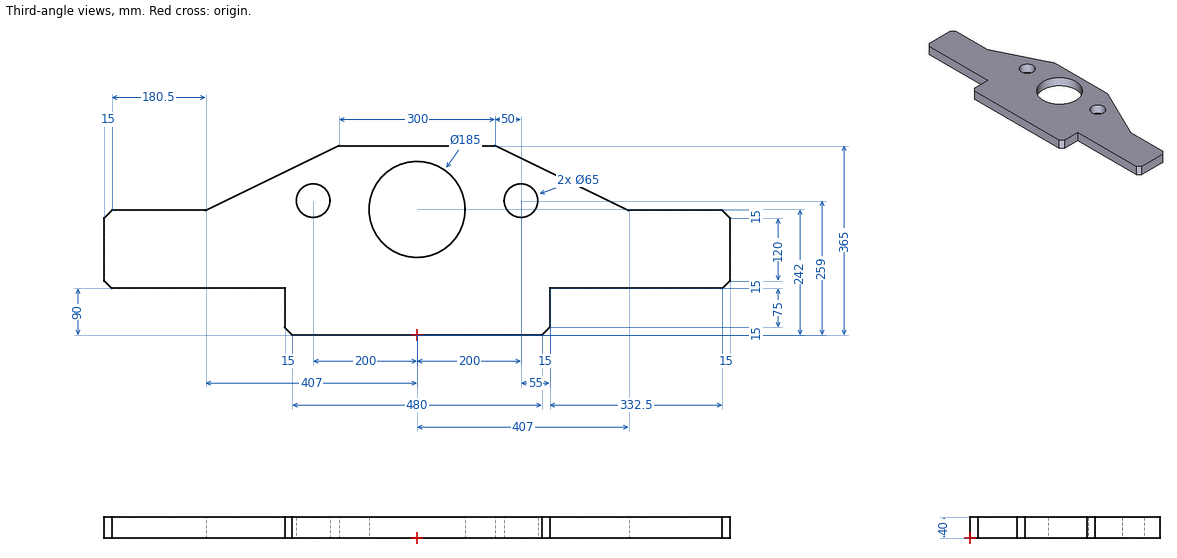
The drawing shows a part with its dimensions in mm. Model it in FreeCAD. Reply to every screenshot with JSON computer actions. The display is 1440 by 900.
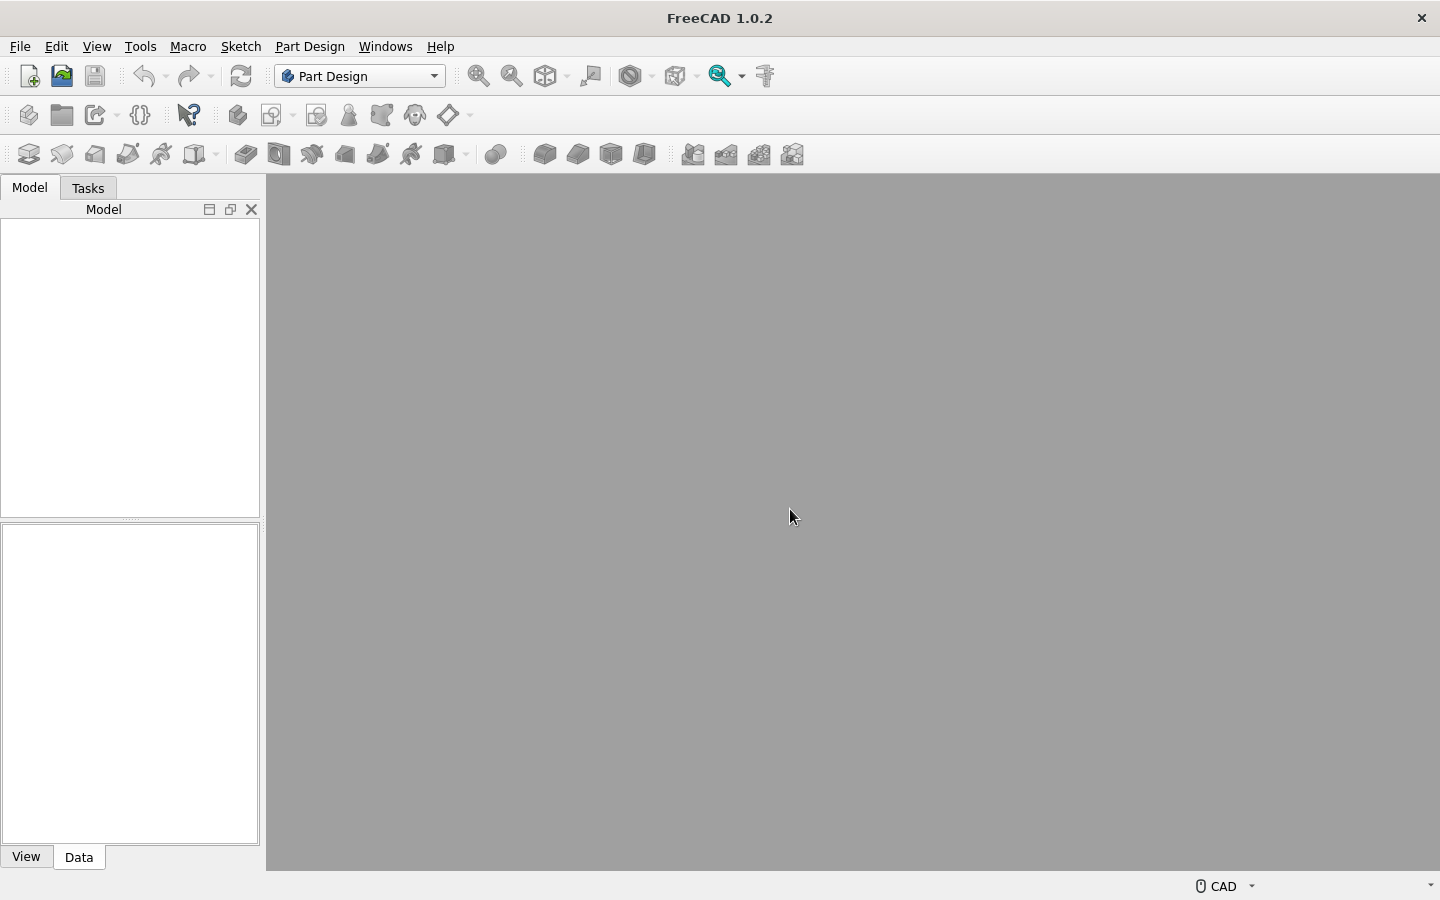
{"action": "left_click", "coordinate": [29, 76]}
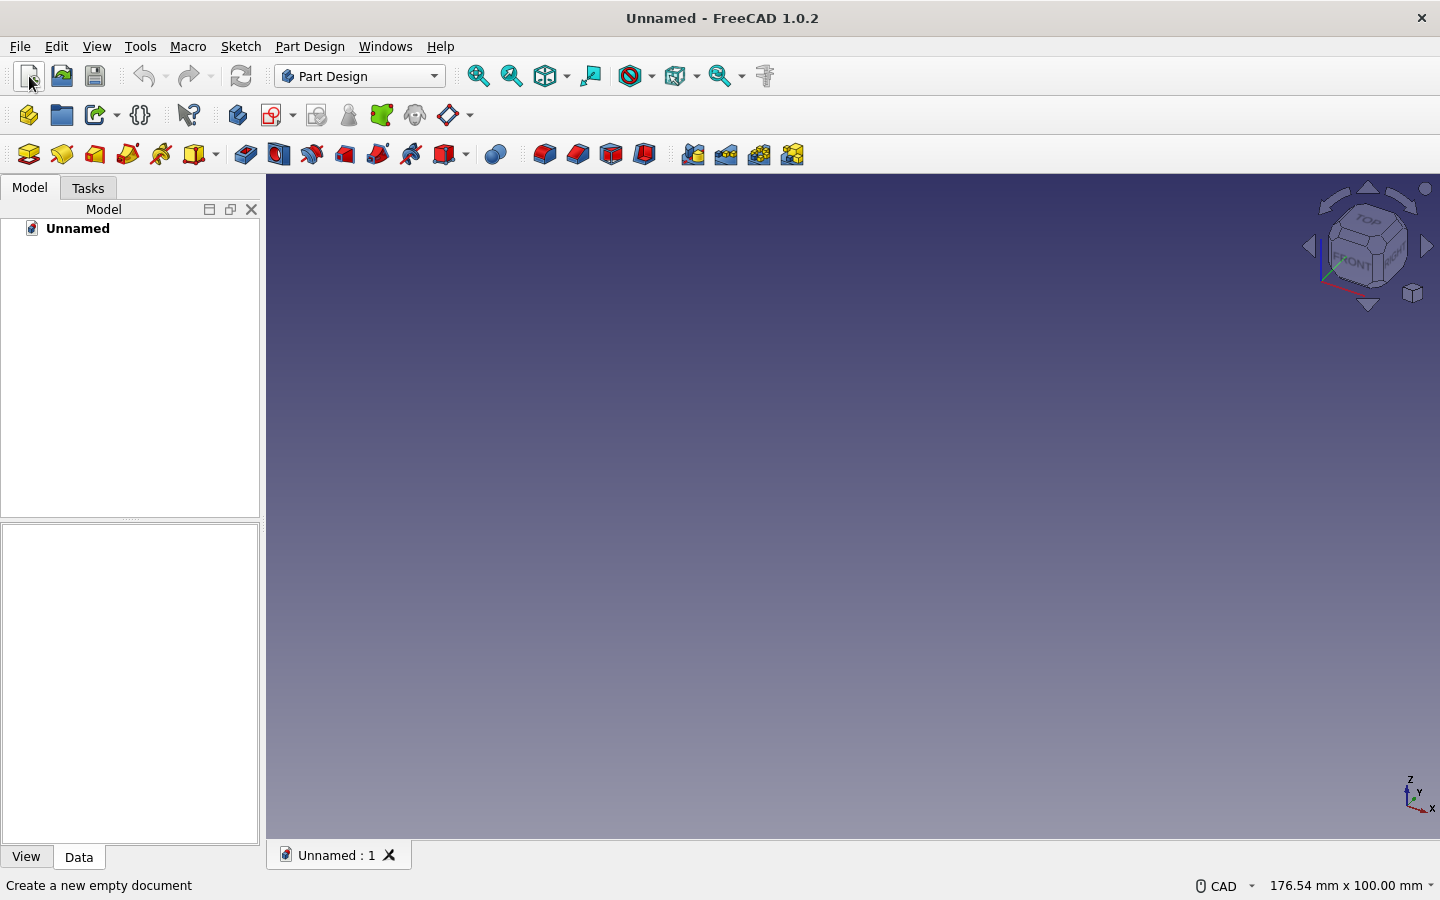
{"action": "left_click", "coordinate": [270, 116]}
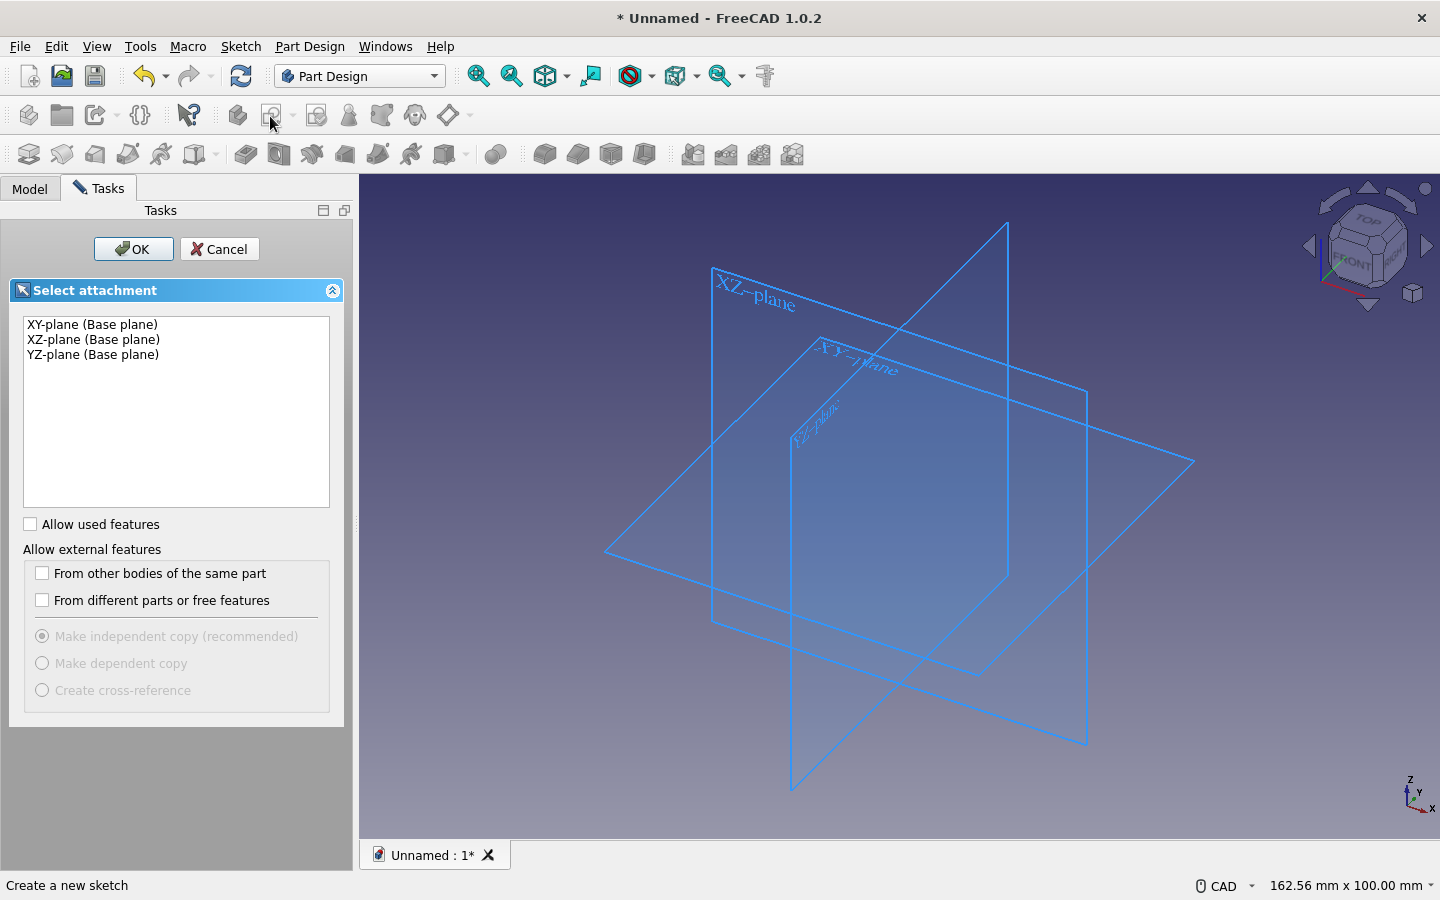
{"action": "left_click", "coordinate": [84, 324]}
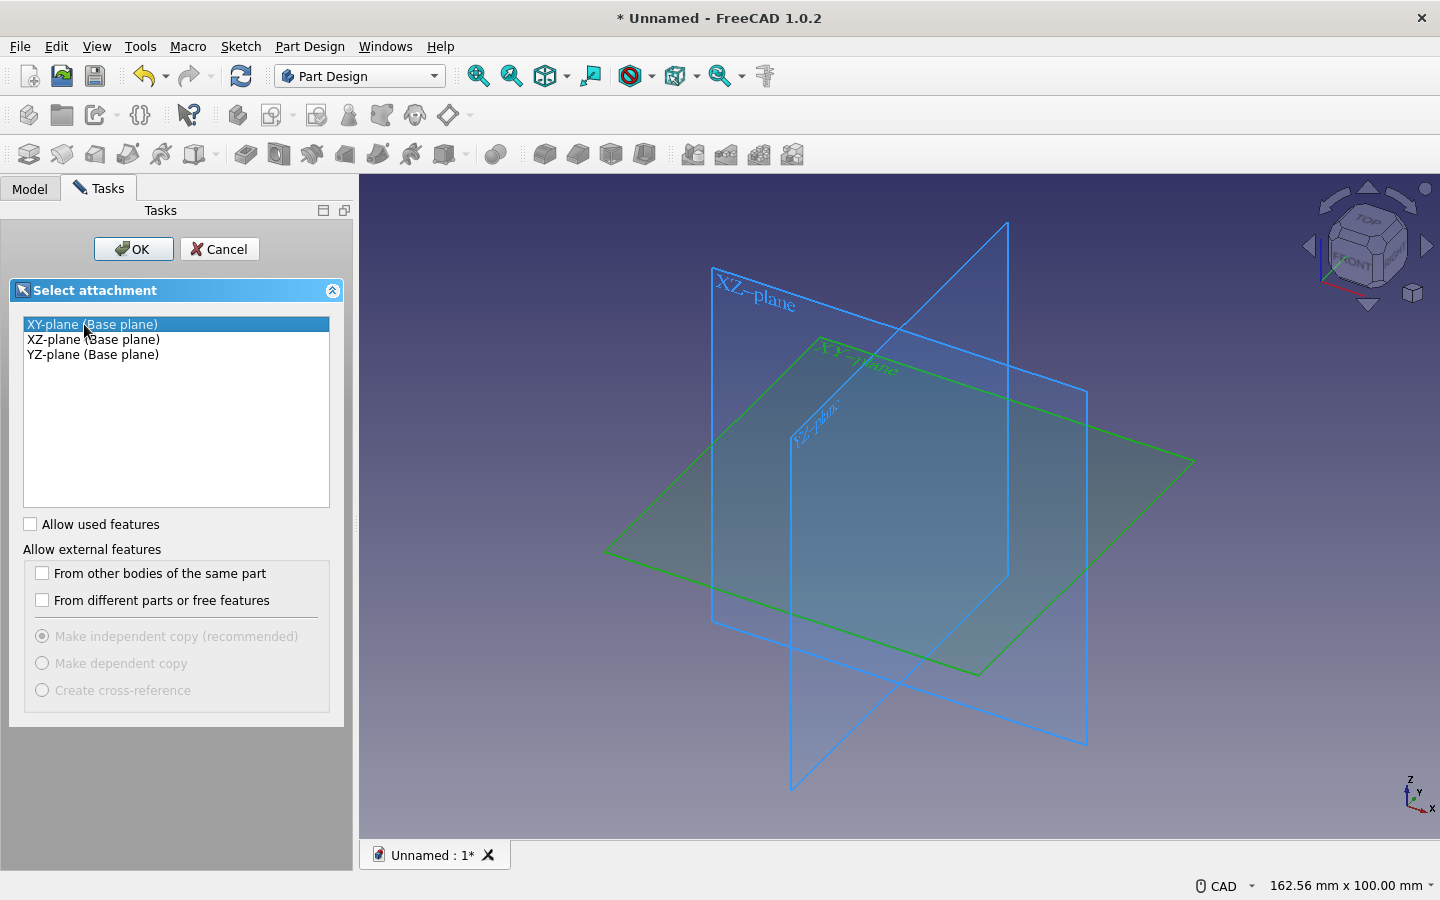
{"action": "left_click", "coordinate": [134, 249]}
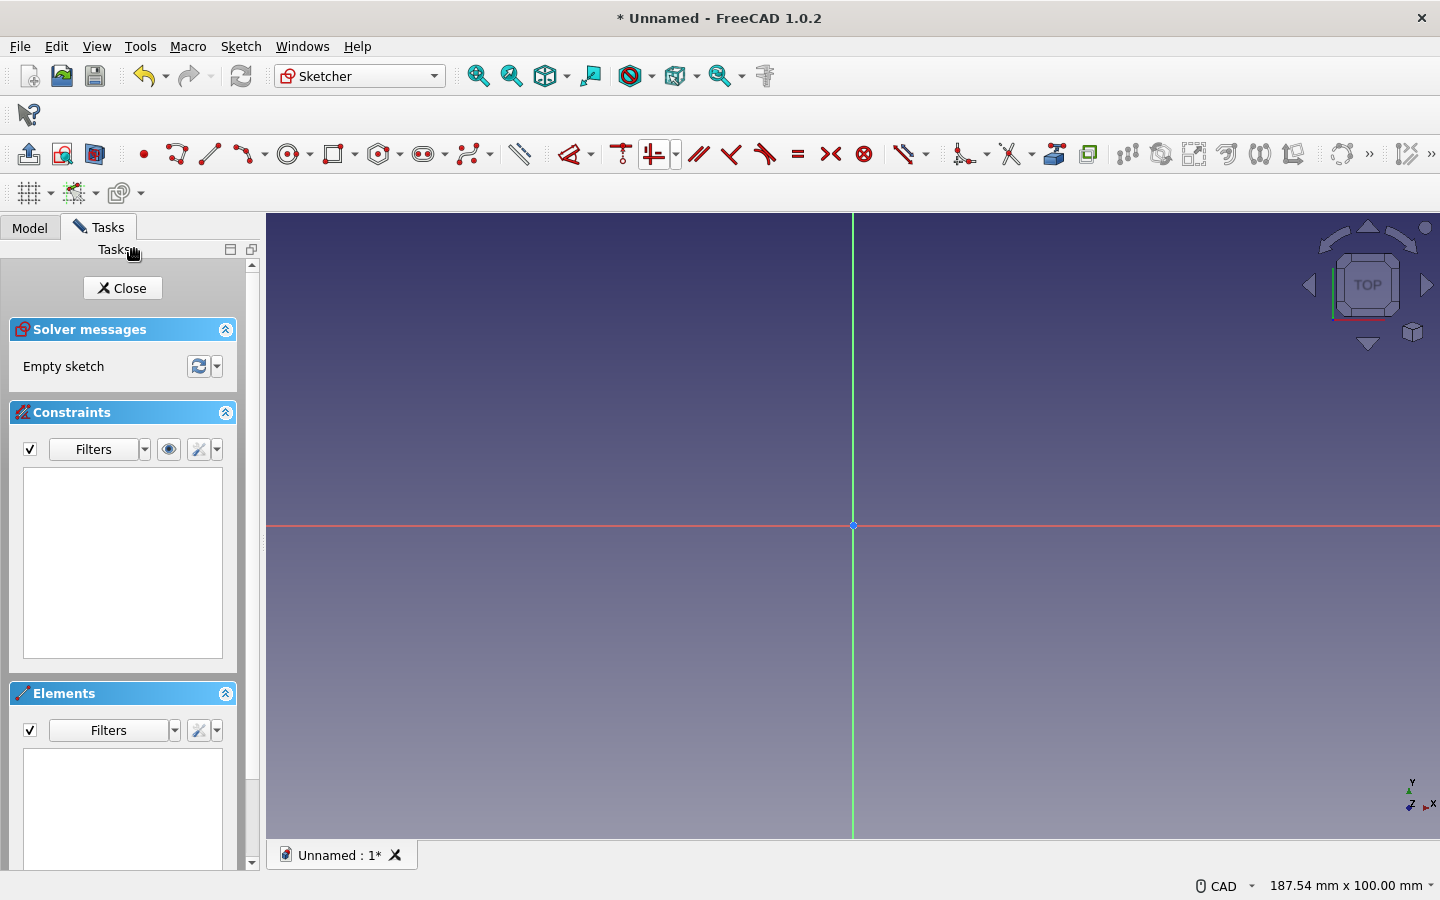
{"action": "scroll", "coordinate": [778, 640], "scroll_direction": "down", "scroll_amount": 12}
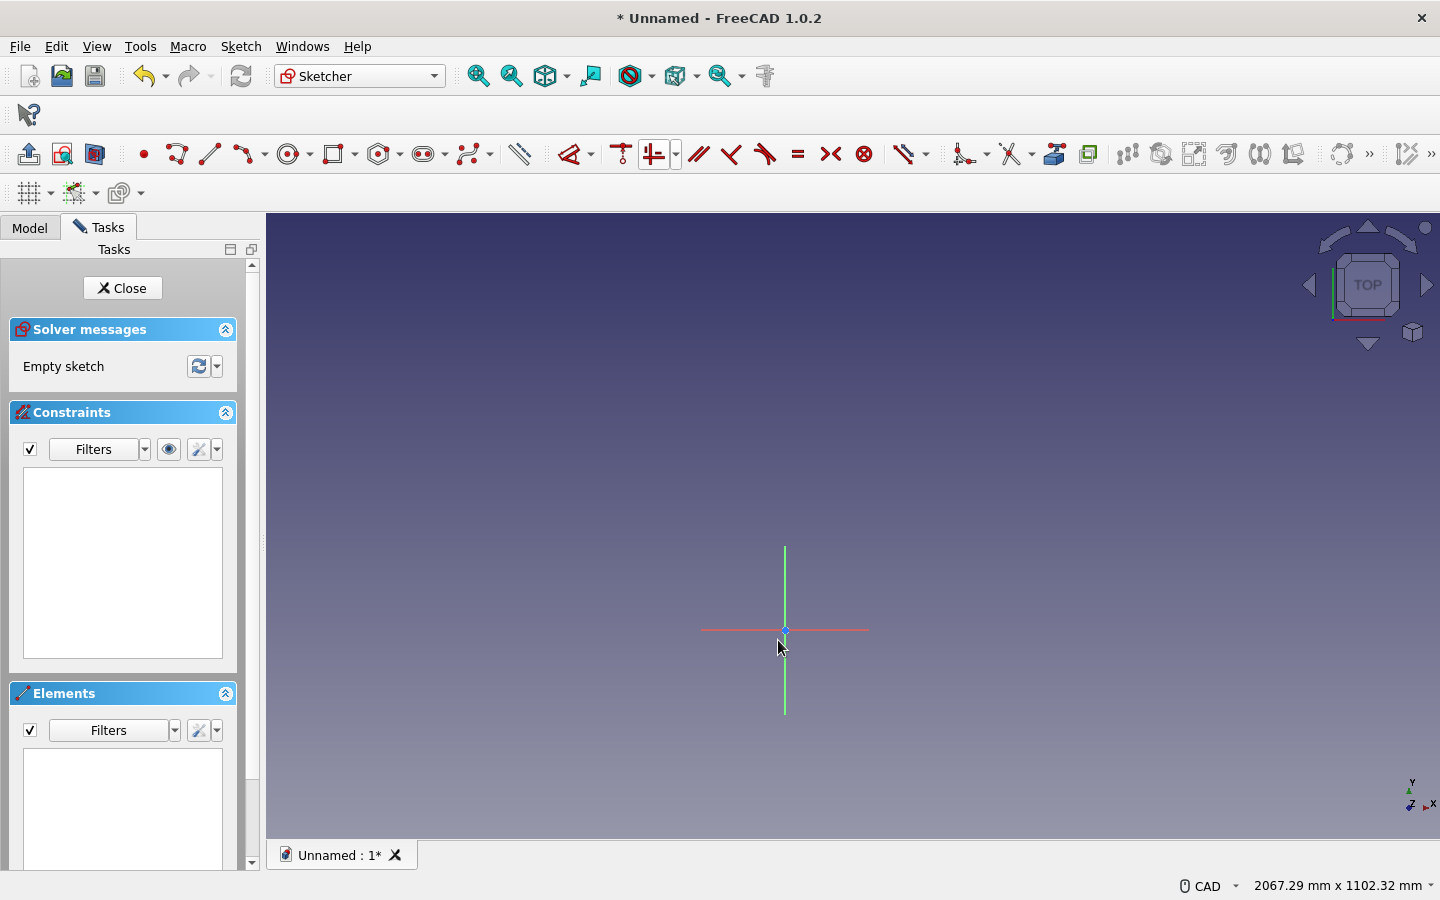
{"action": "left_click", "coordinate": [177, 154]}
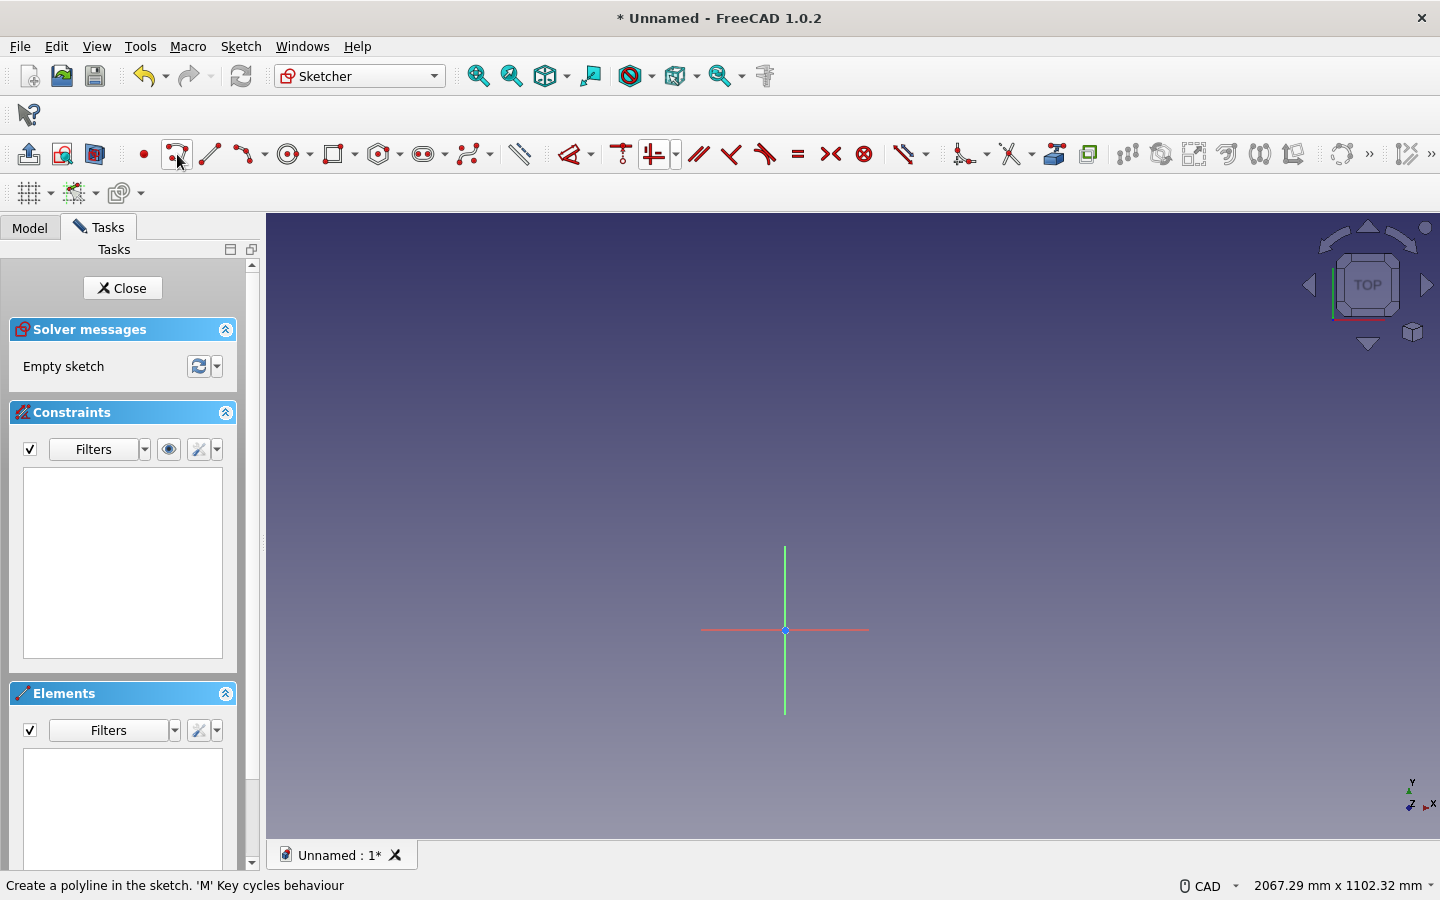
{"action": "left_click", "coordinate": [649, 630]}
{"action": "left_click", "coordinate": [921, 621]}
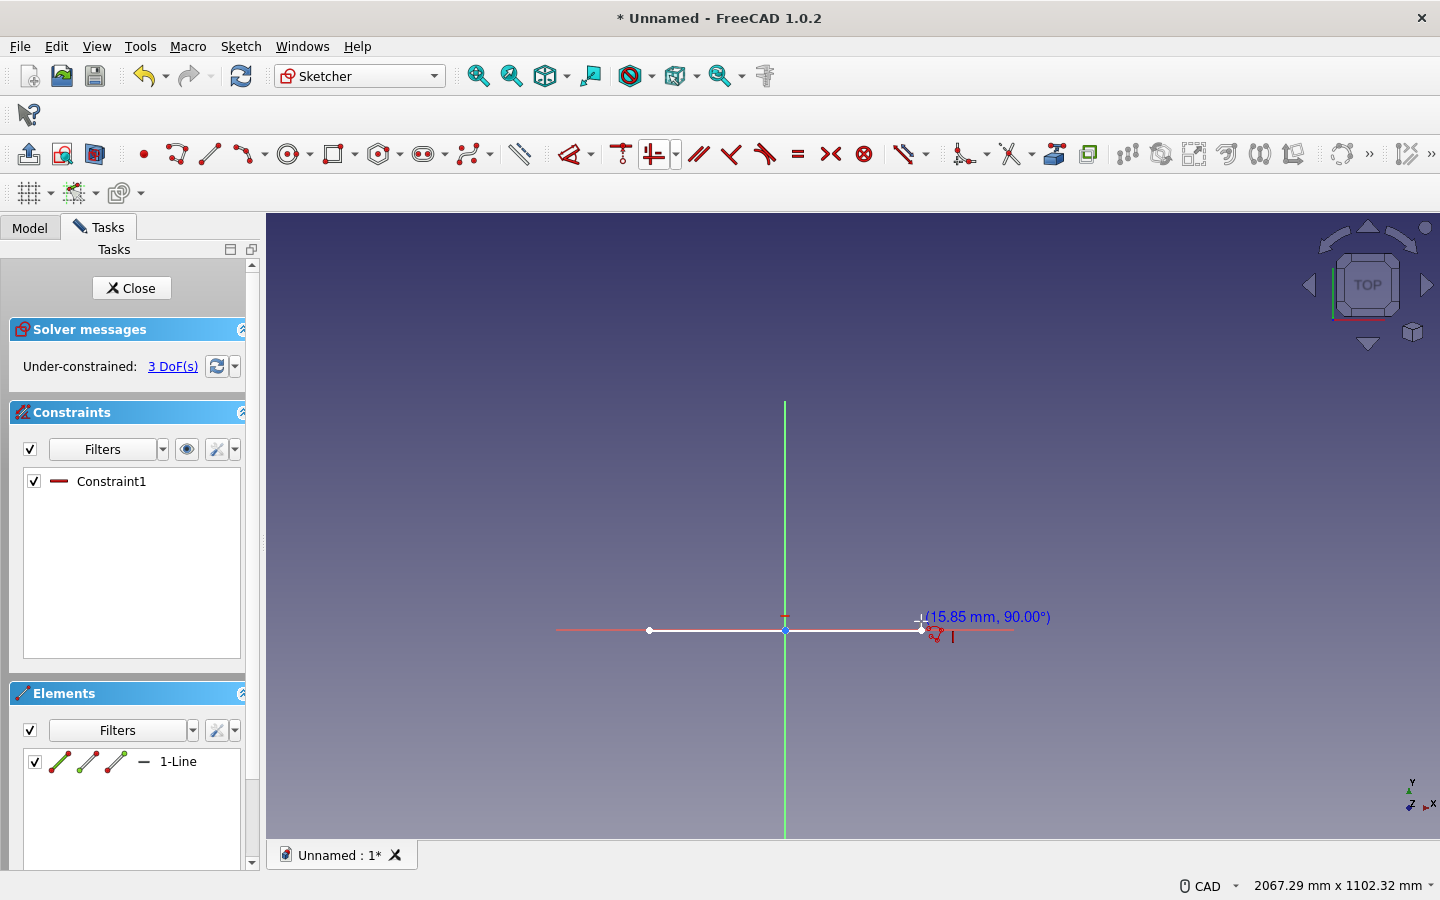
{"action": "scroll", "coordinate": [930, 622], "scroll_direction": "up", "scroll_amount": 4}